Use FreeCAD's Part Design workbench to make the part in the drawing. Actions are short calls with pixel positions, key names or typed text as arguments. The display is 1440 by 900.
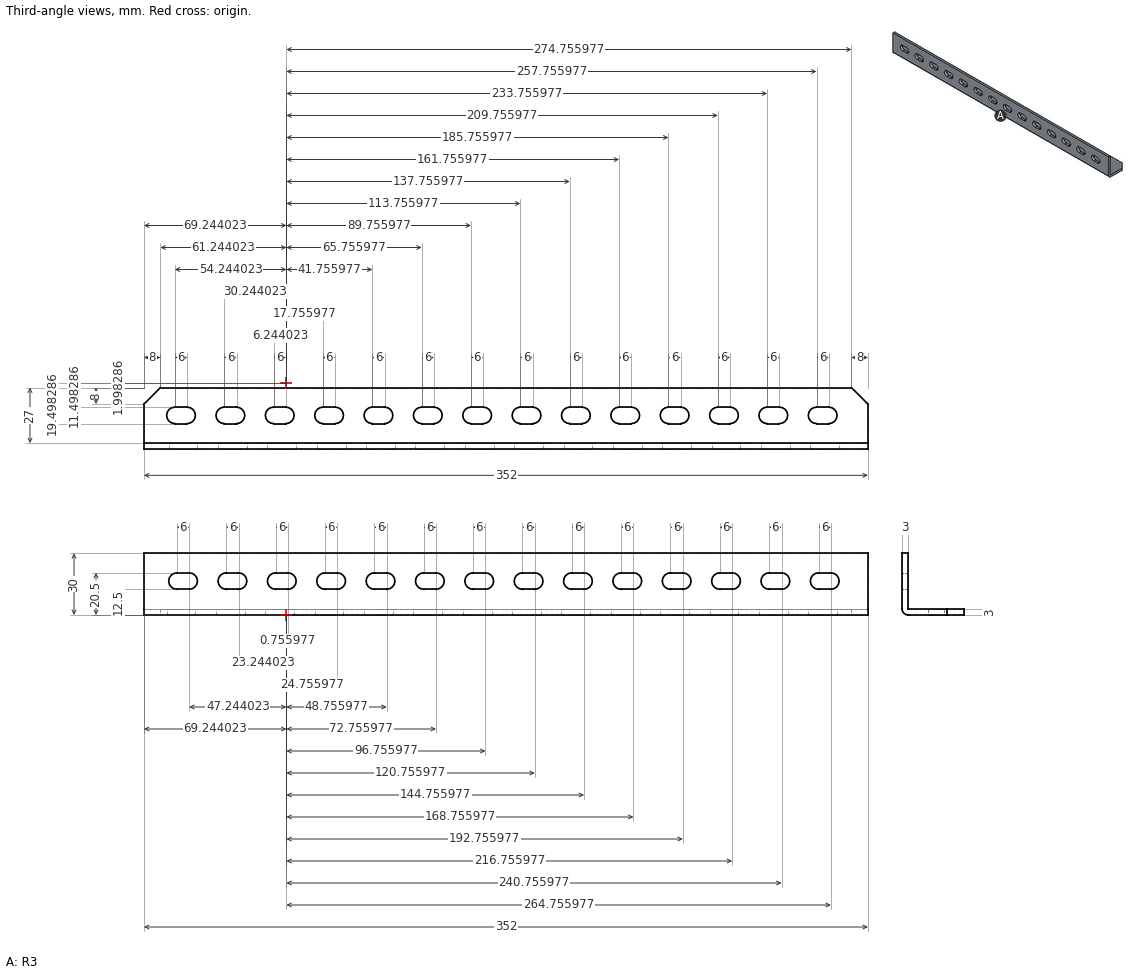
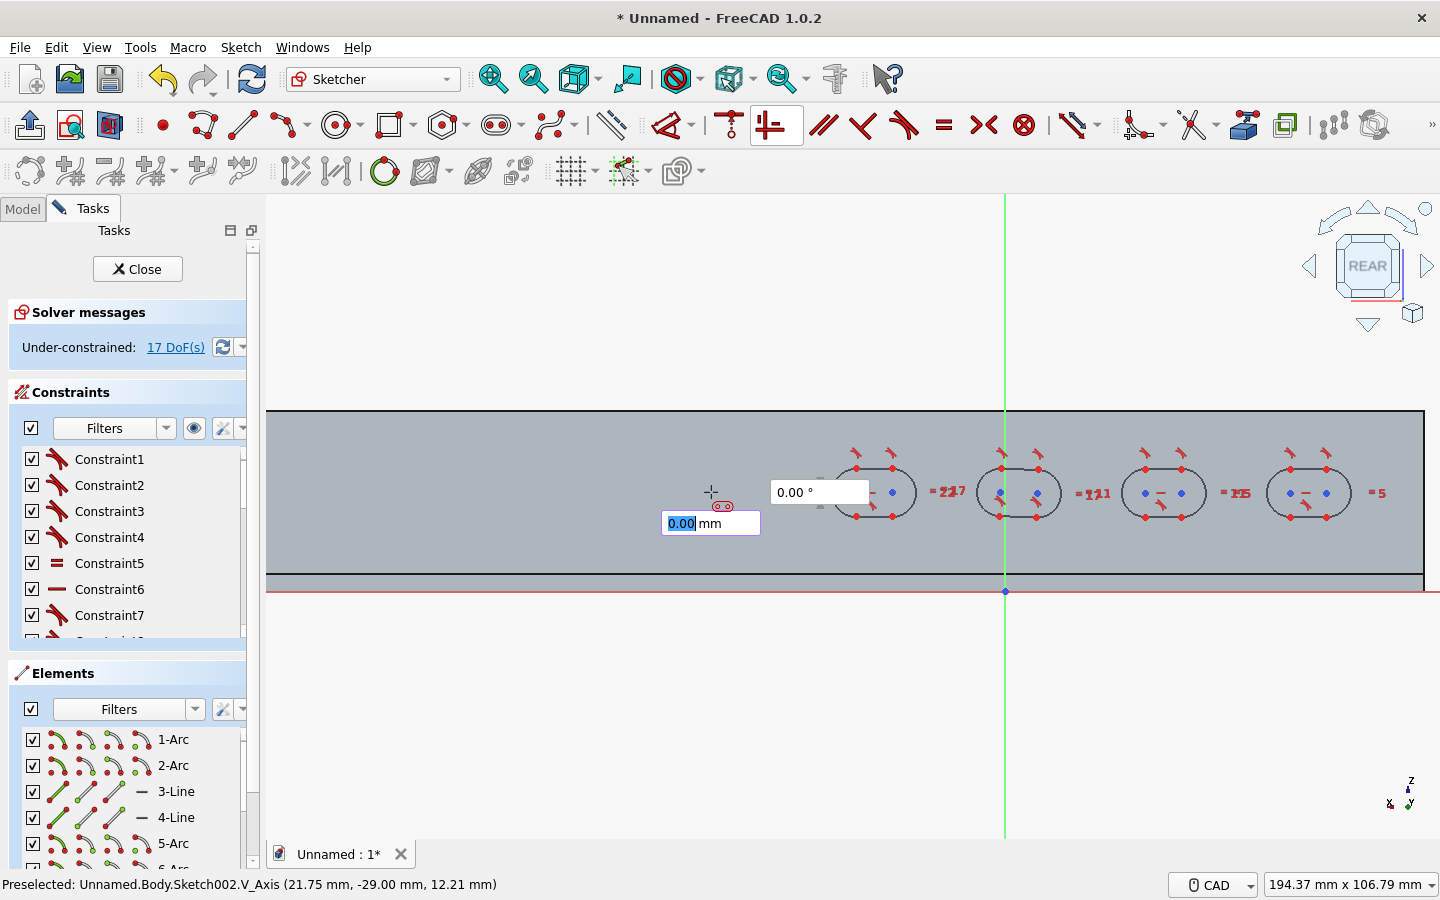
click(747, 492)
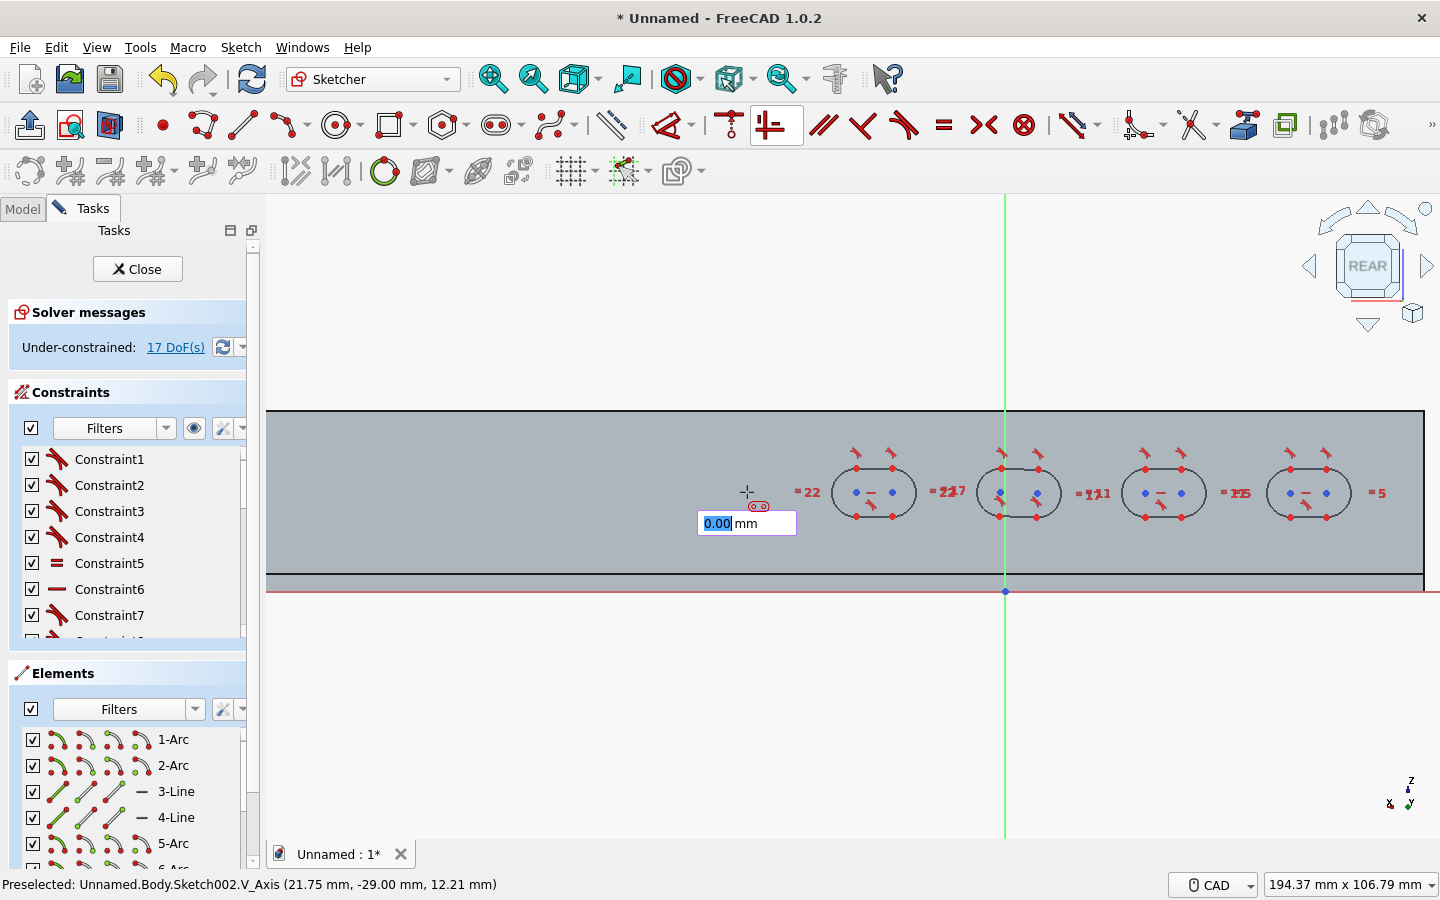
click(729, 516)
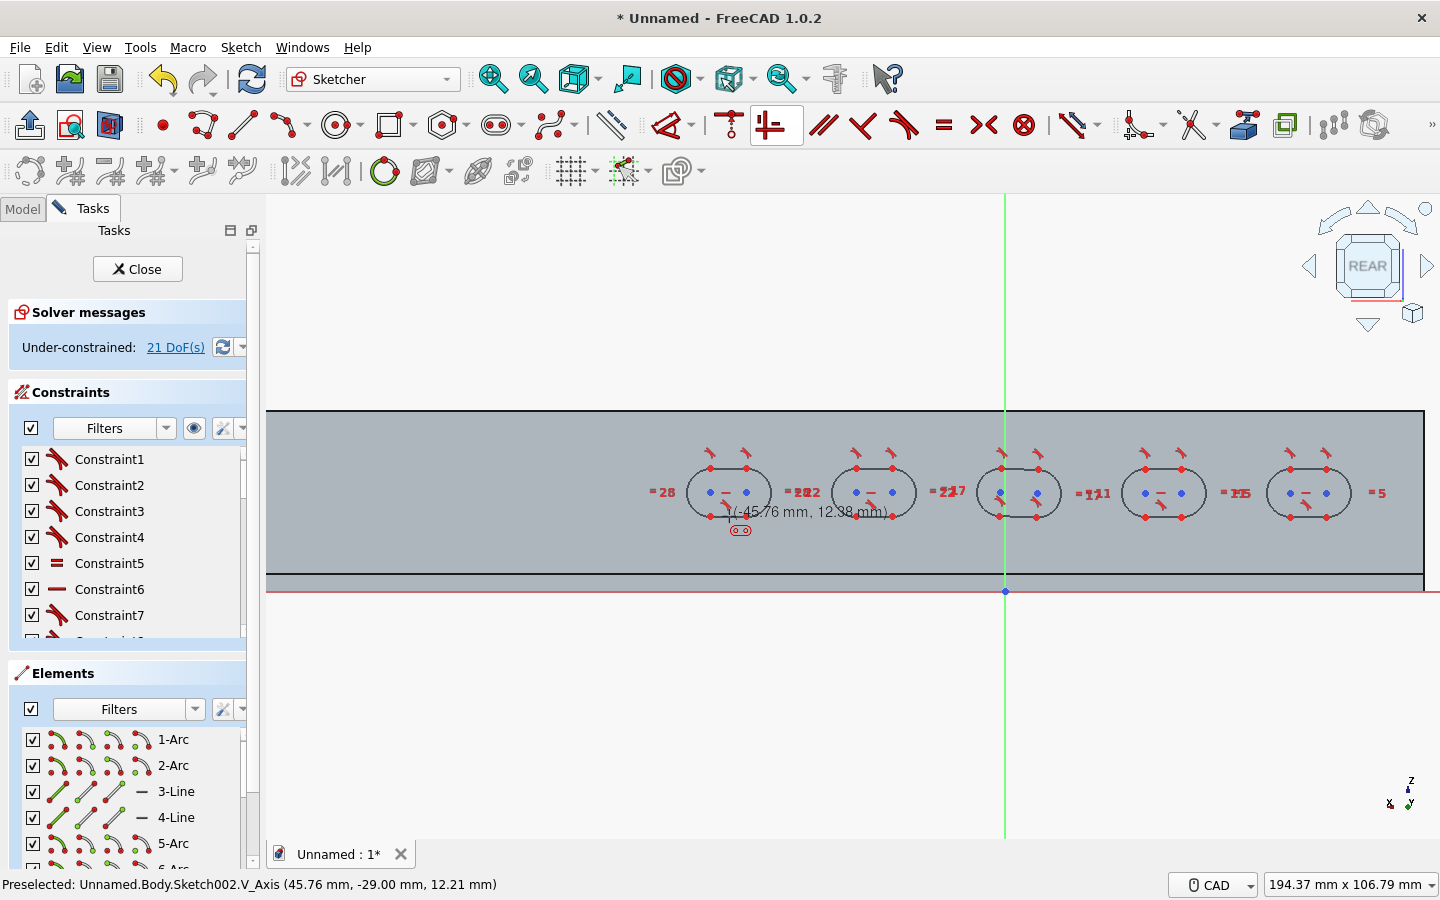
click(566, 492)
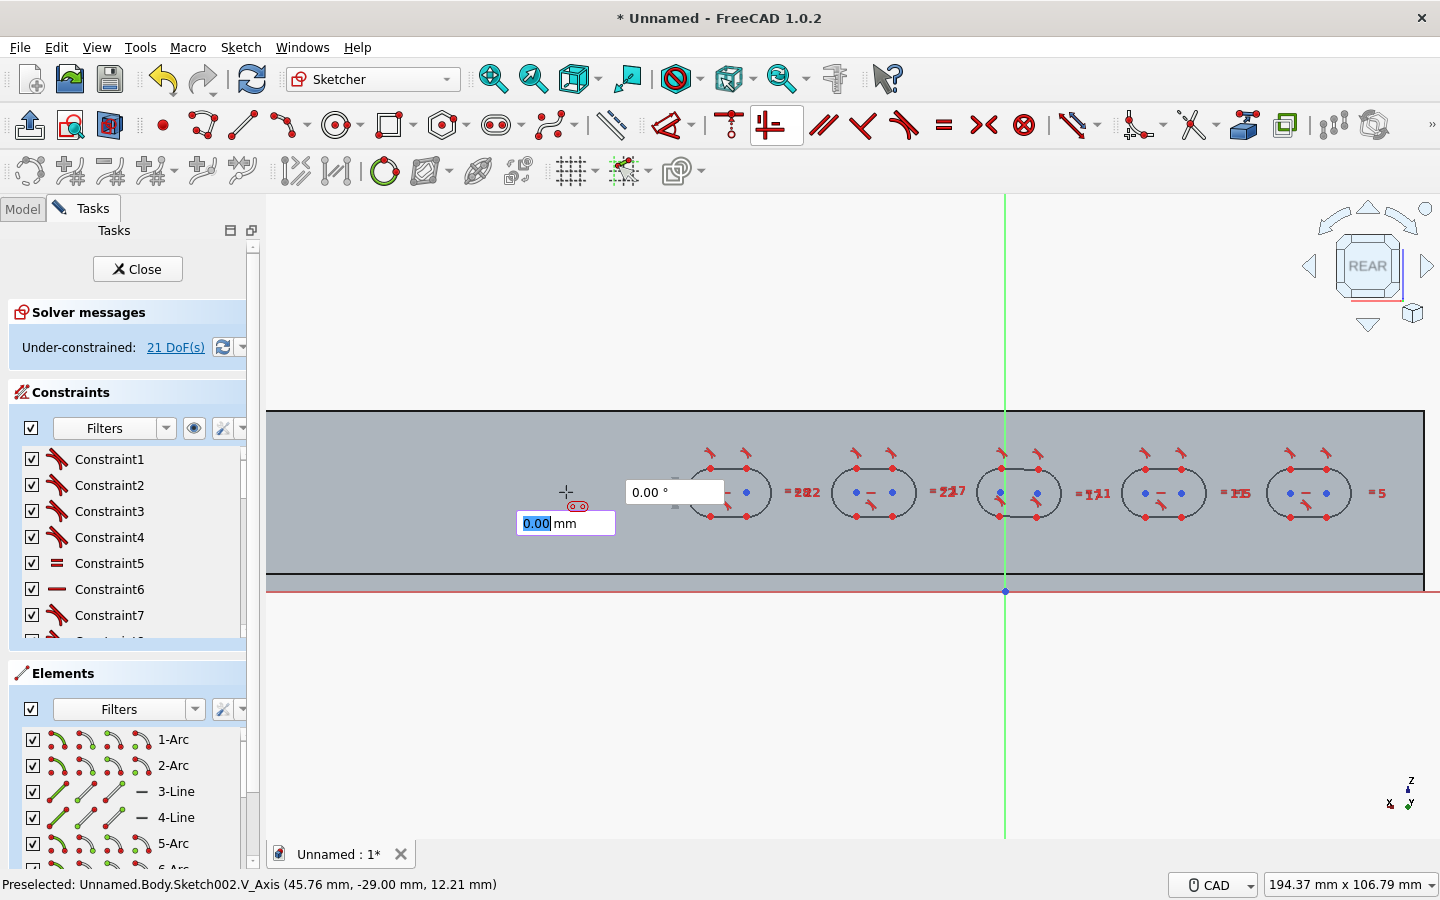
click(602, 492)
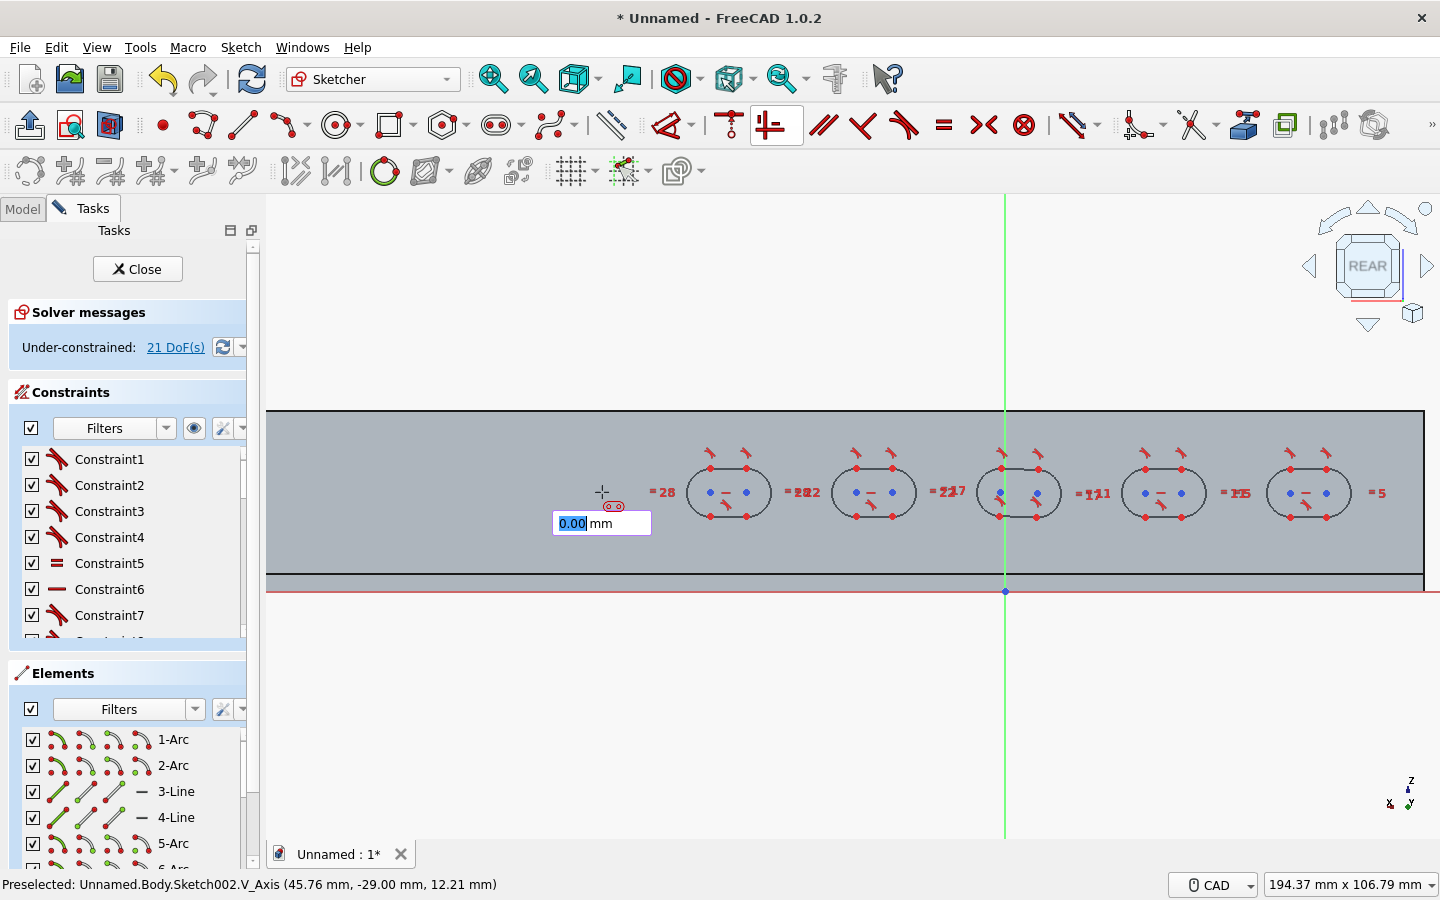
click(584, 516)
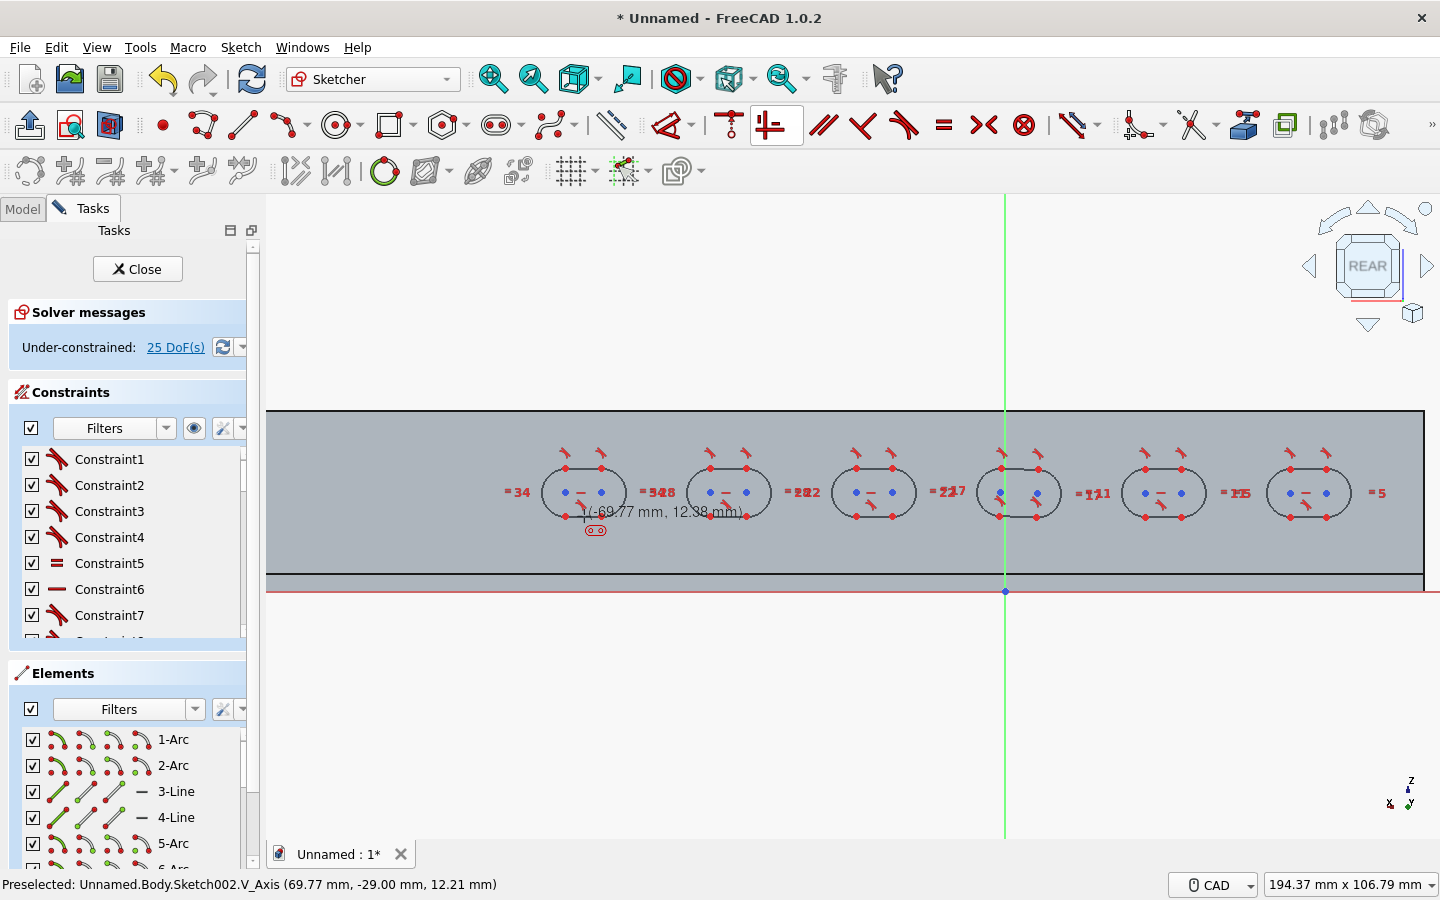
click(421, 492)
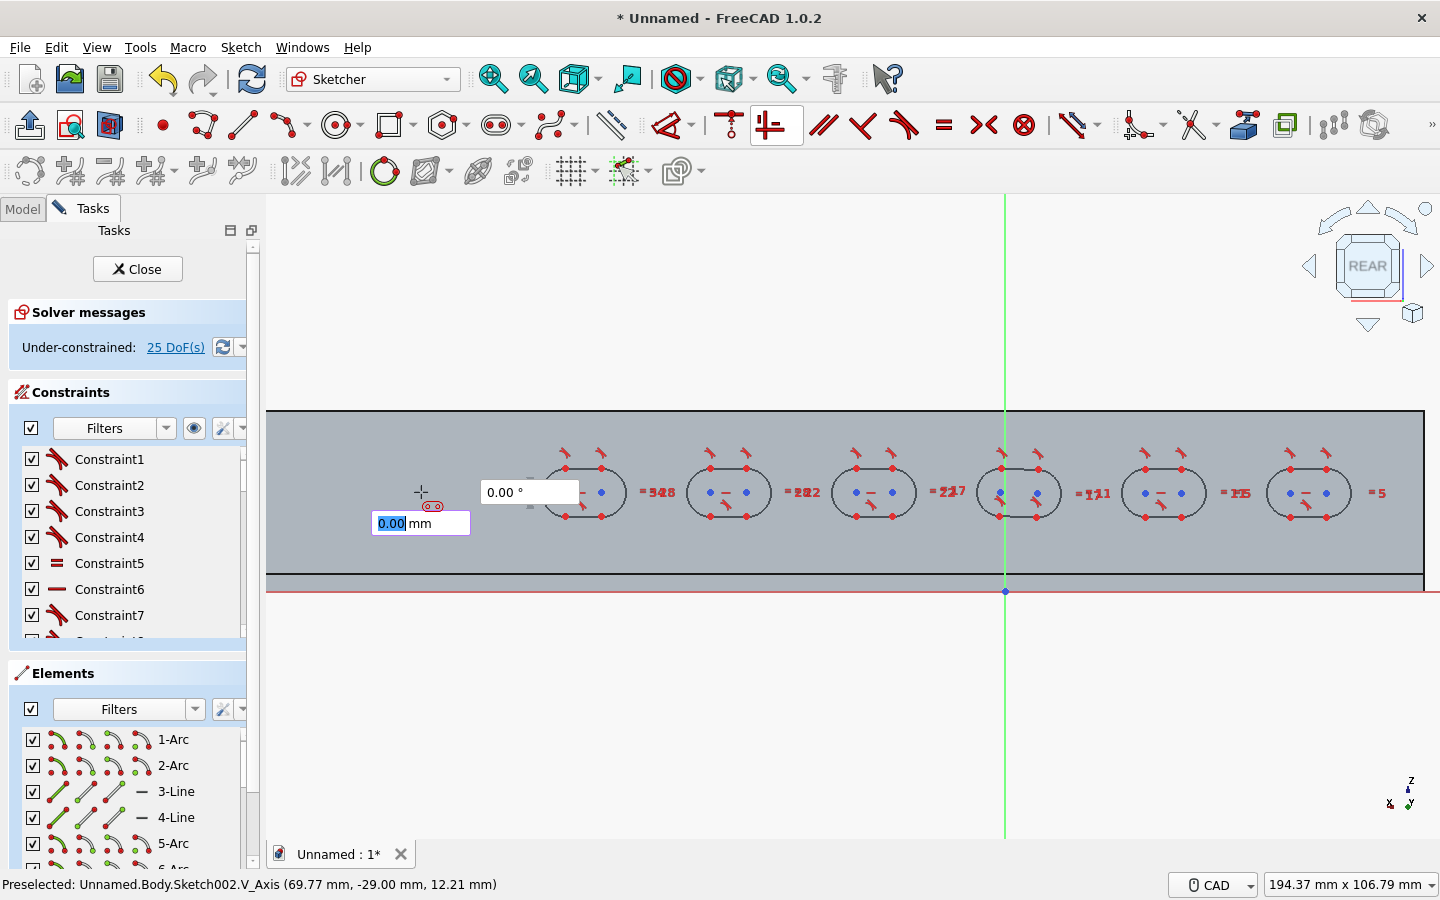
click(457, 492)